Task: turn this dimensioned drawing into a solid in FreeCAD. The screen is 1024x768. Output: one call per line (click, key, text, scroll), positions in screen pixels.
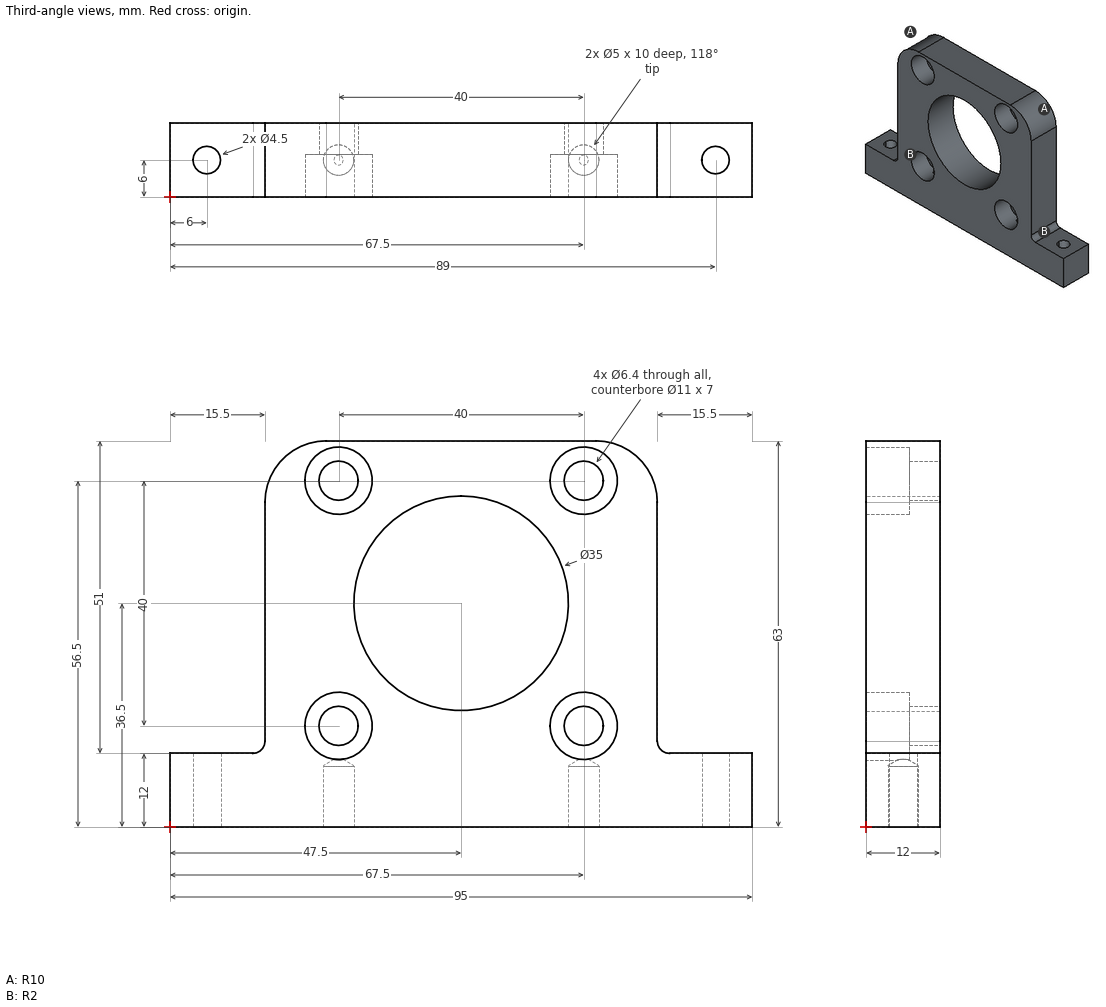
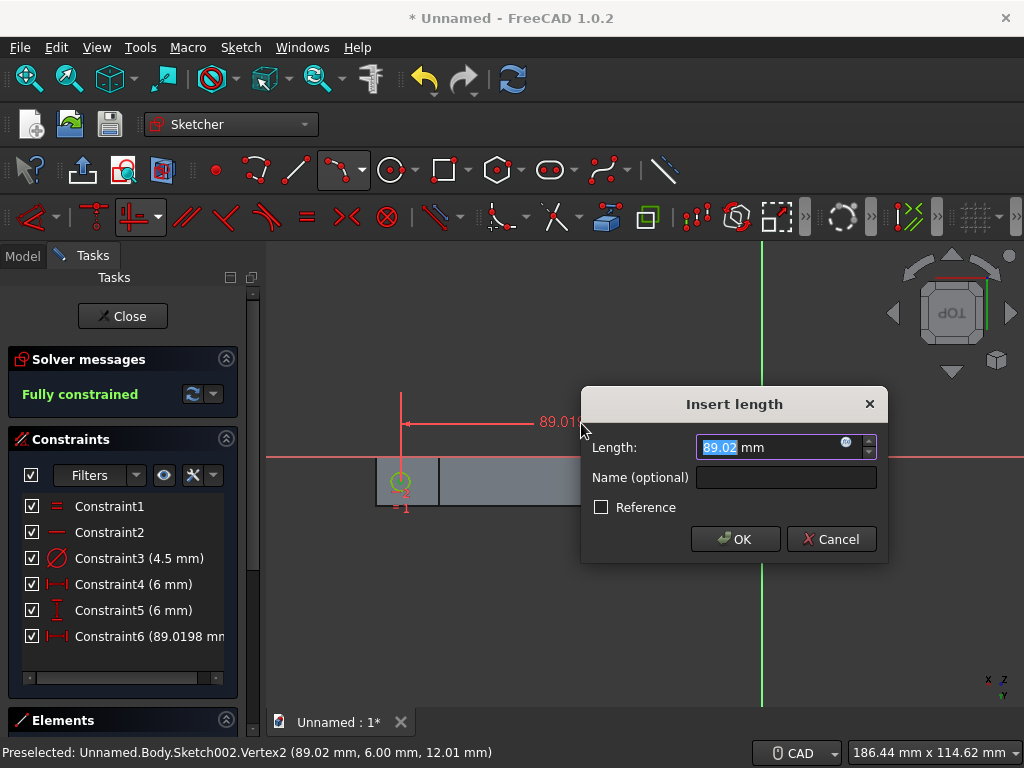
text(89)
key(Return)
key(Escape)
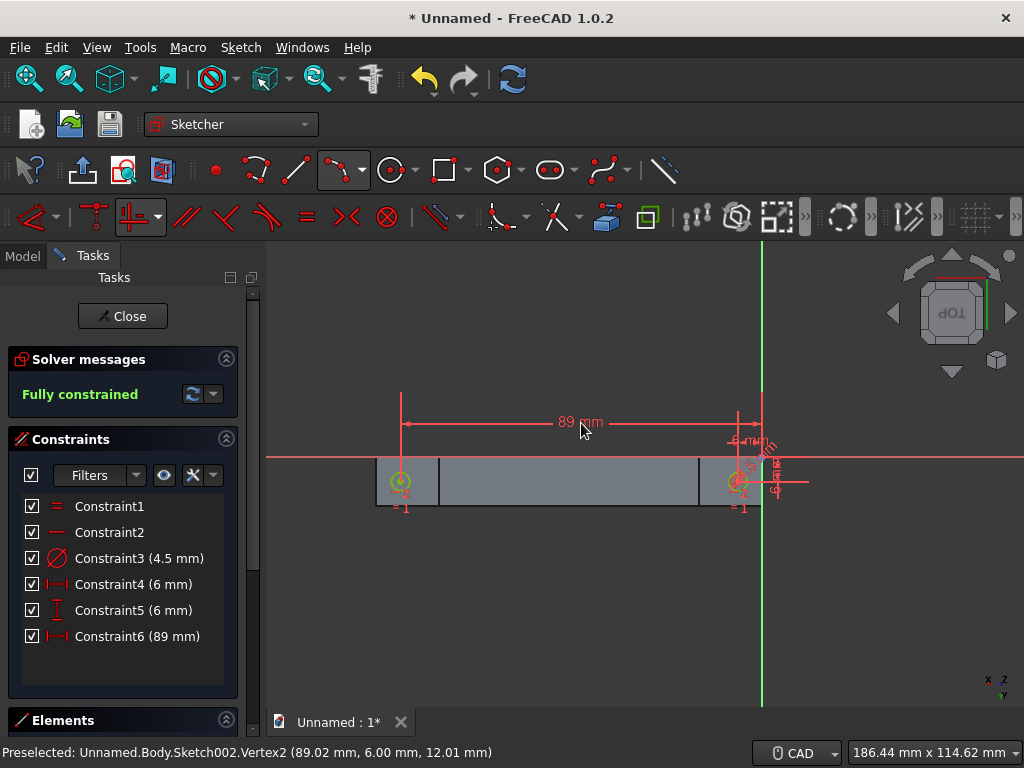
click(123, 316)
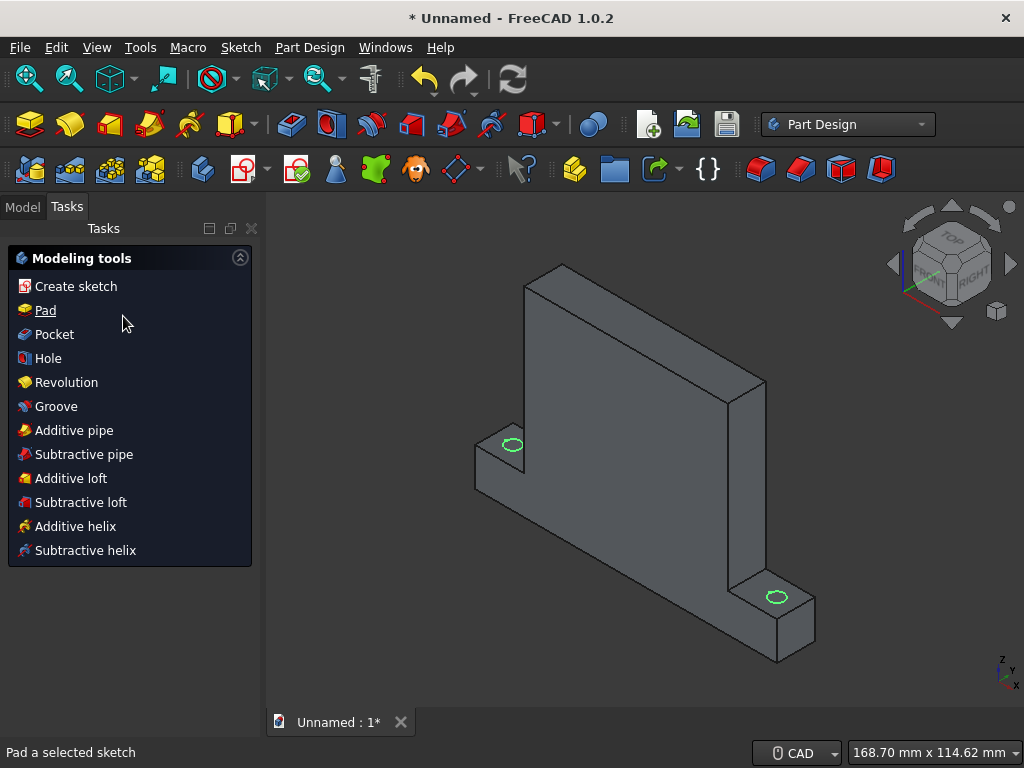
click(292, 124)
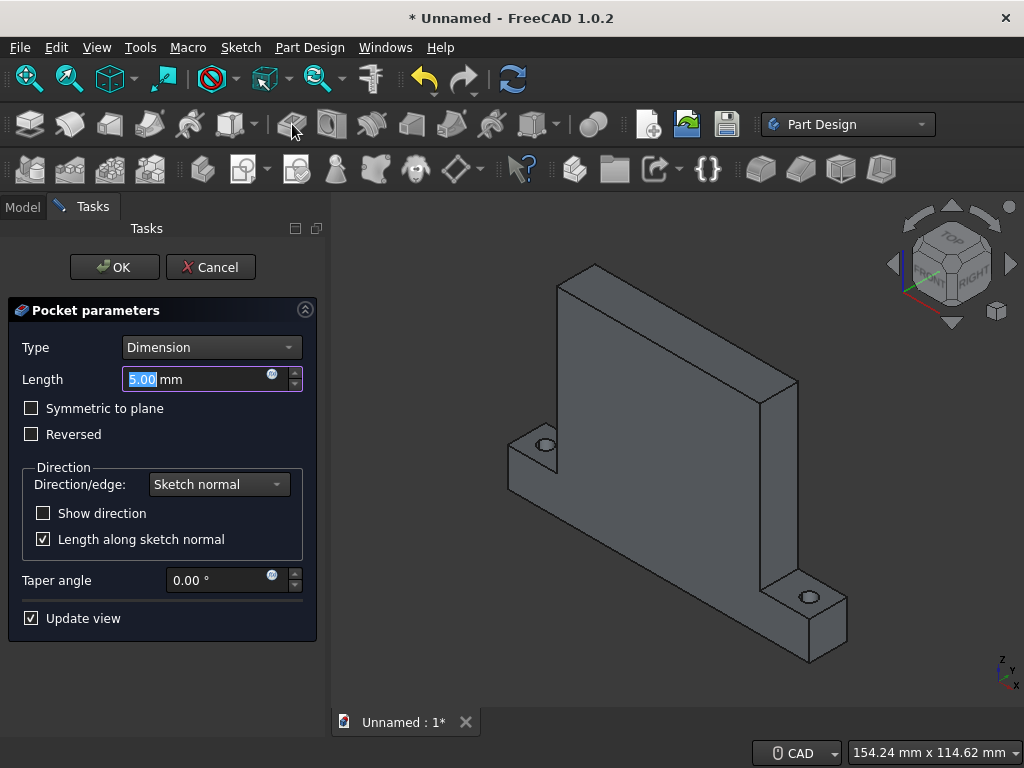
click(212, 348)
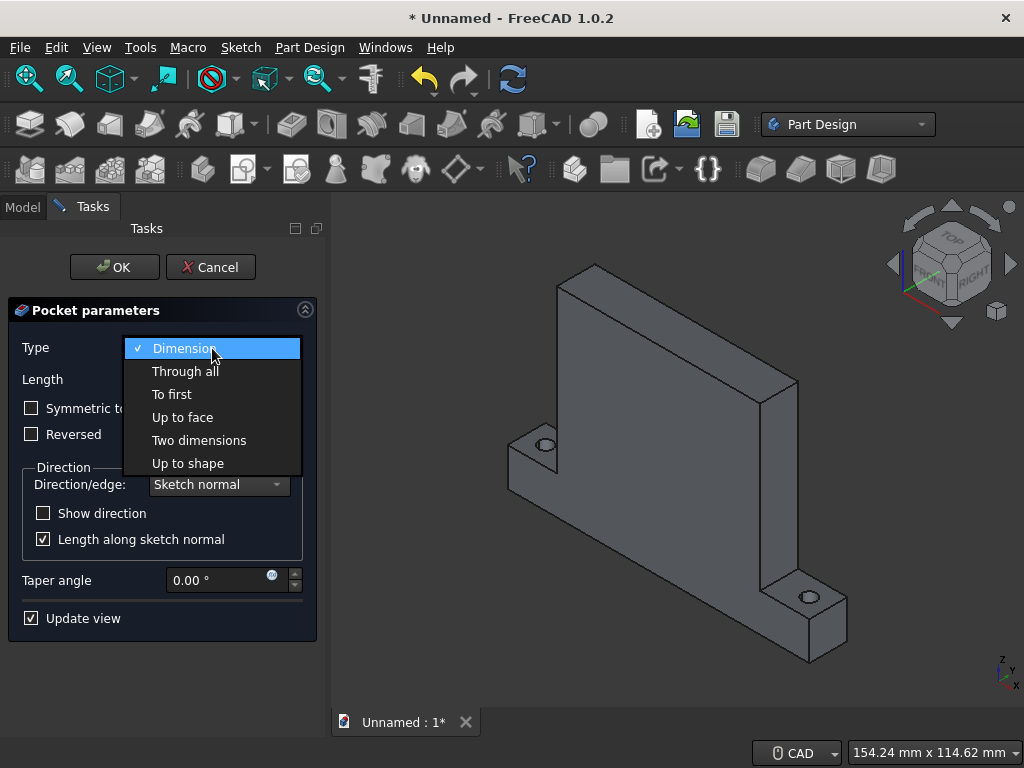
click(212, 372)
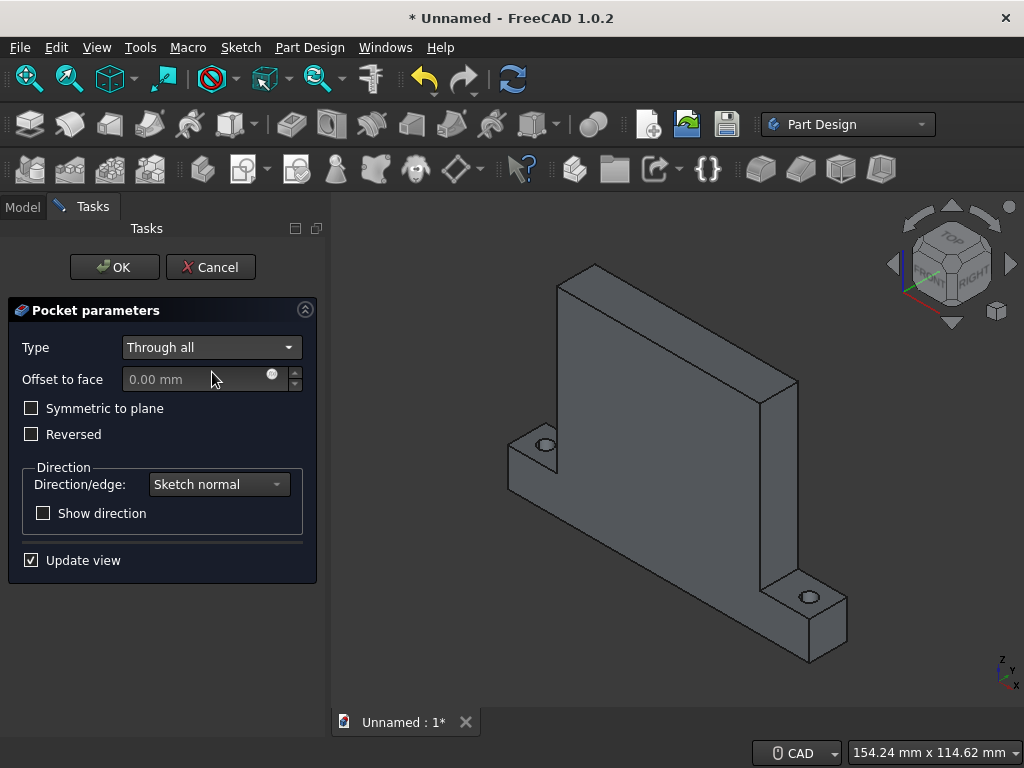
click(115, 267)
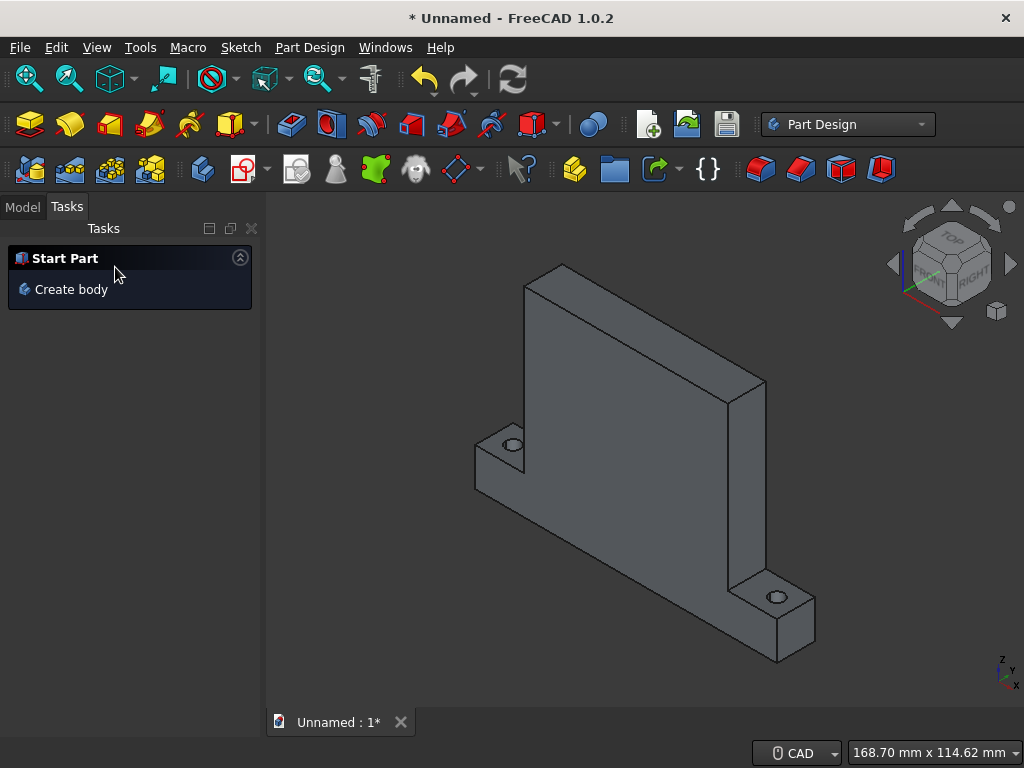
key(4)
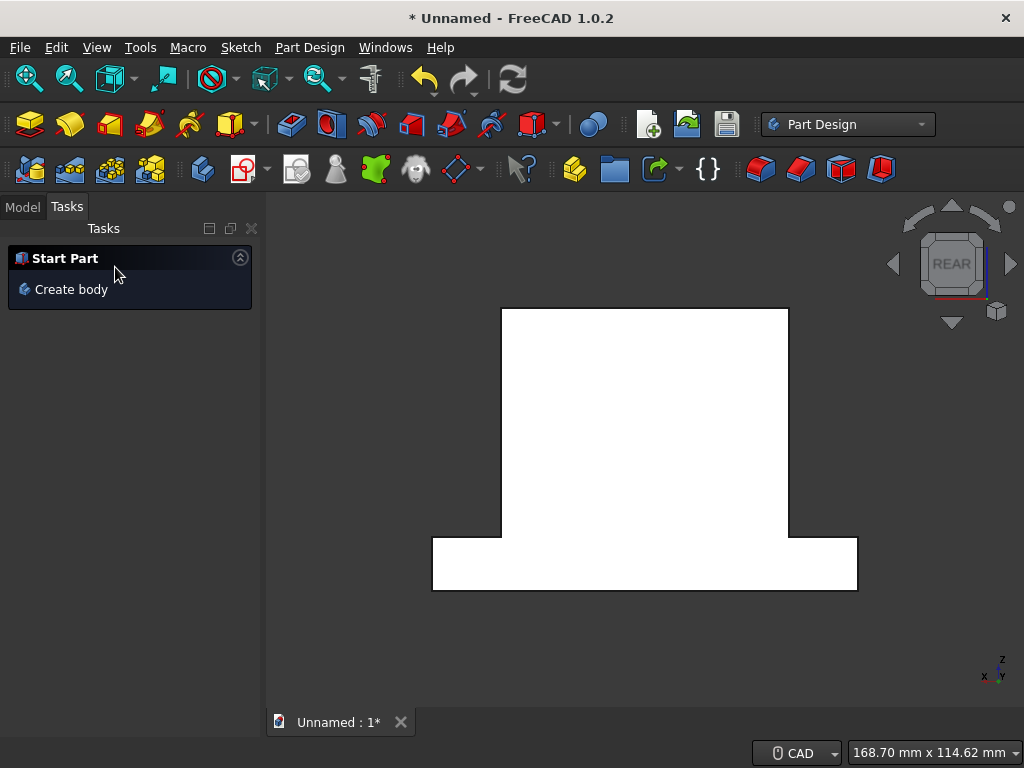
click(645, 449)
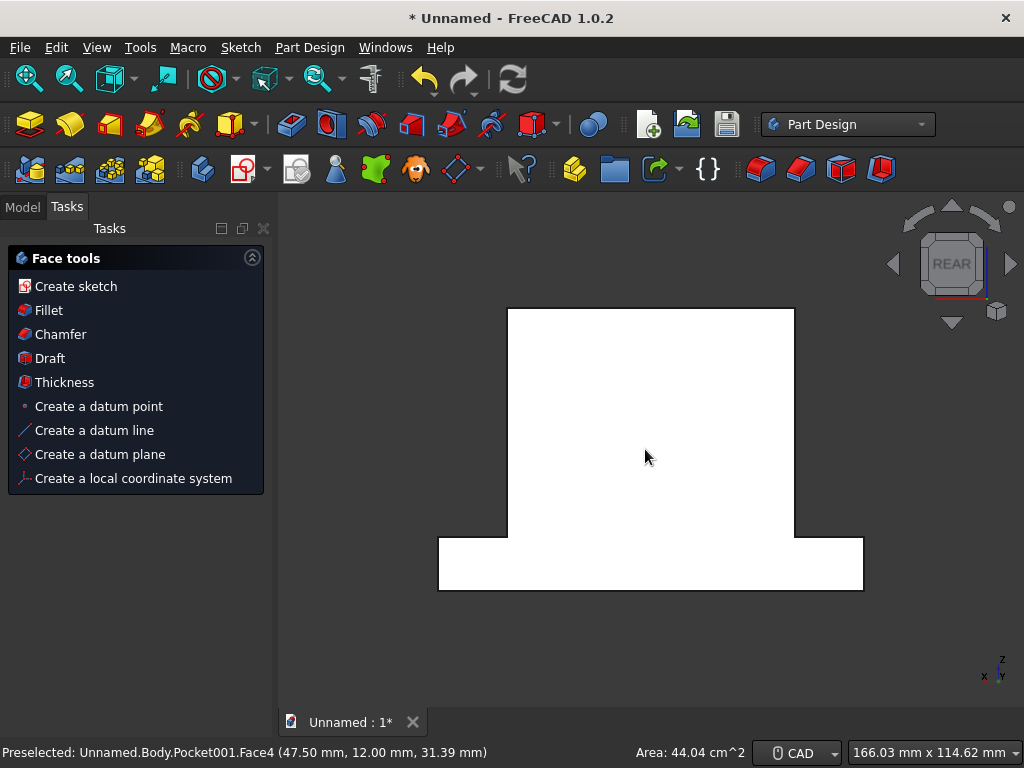
click(244, 170)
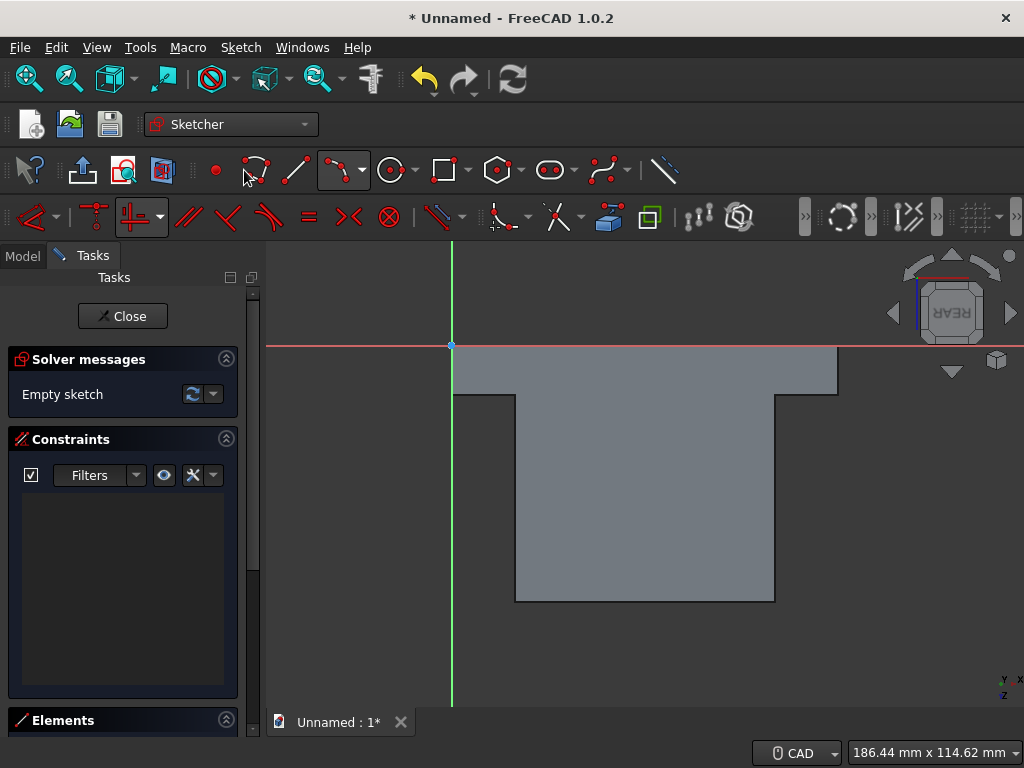
click(392, 170)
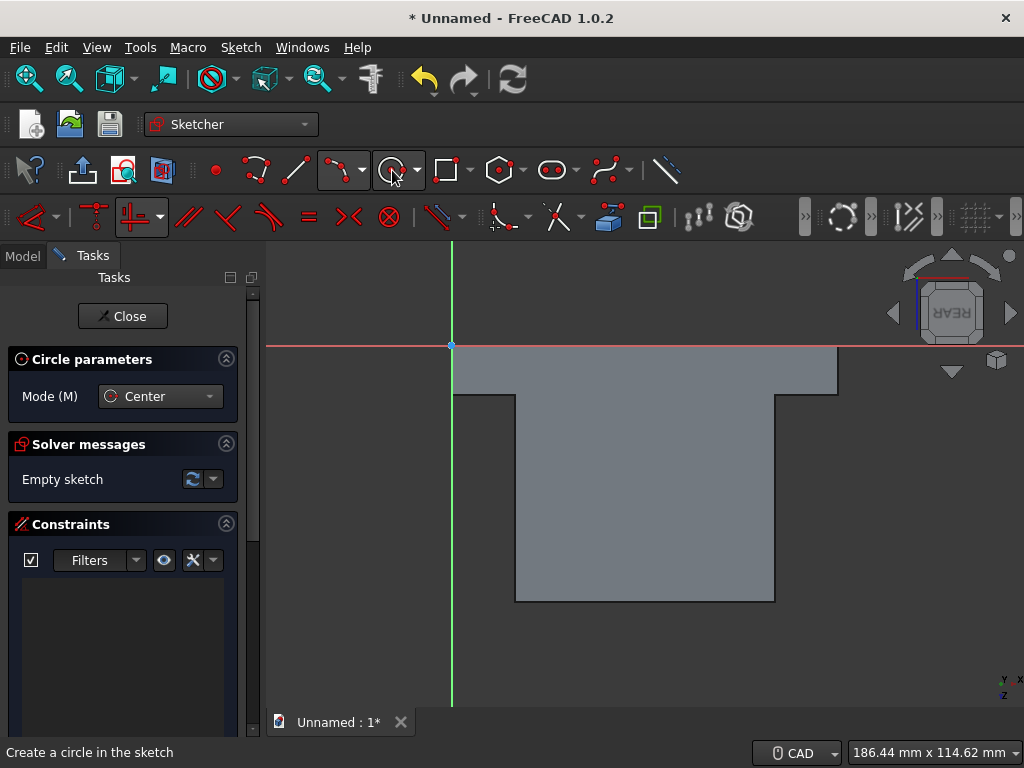
click(645, 494)
click(695, 444)
key(Escape)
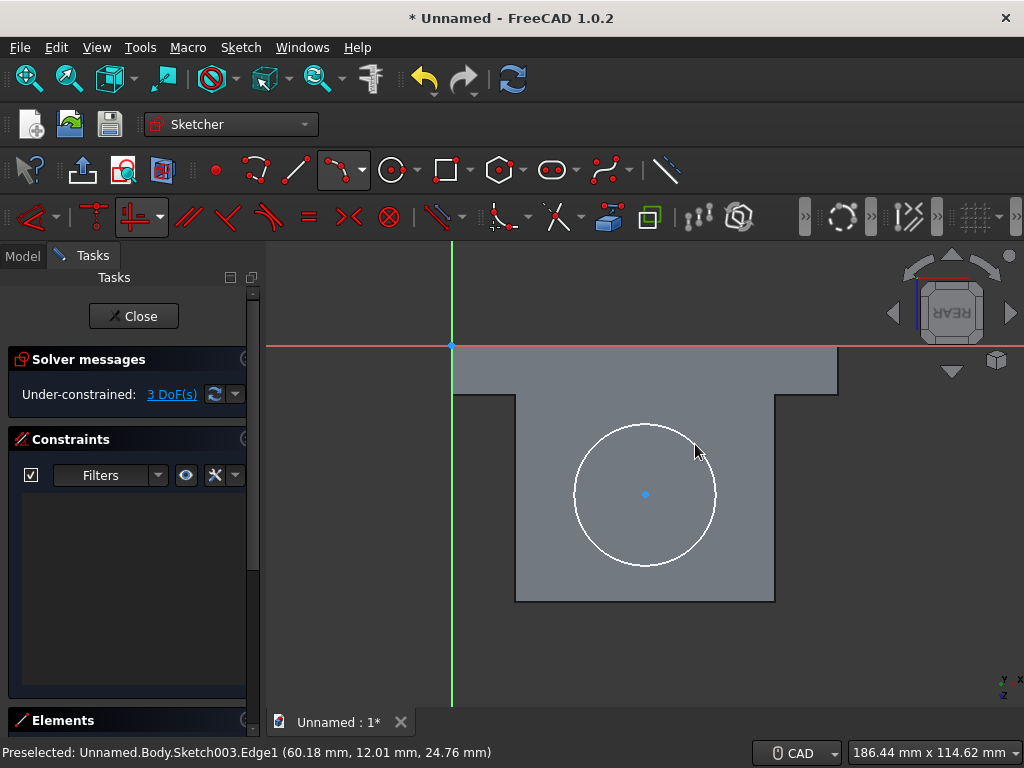
key(d)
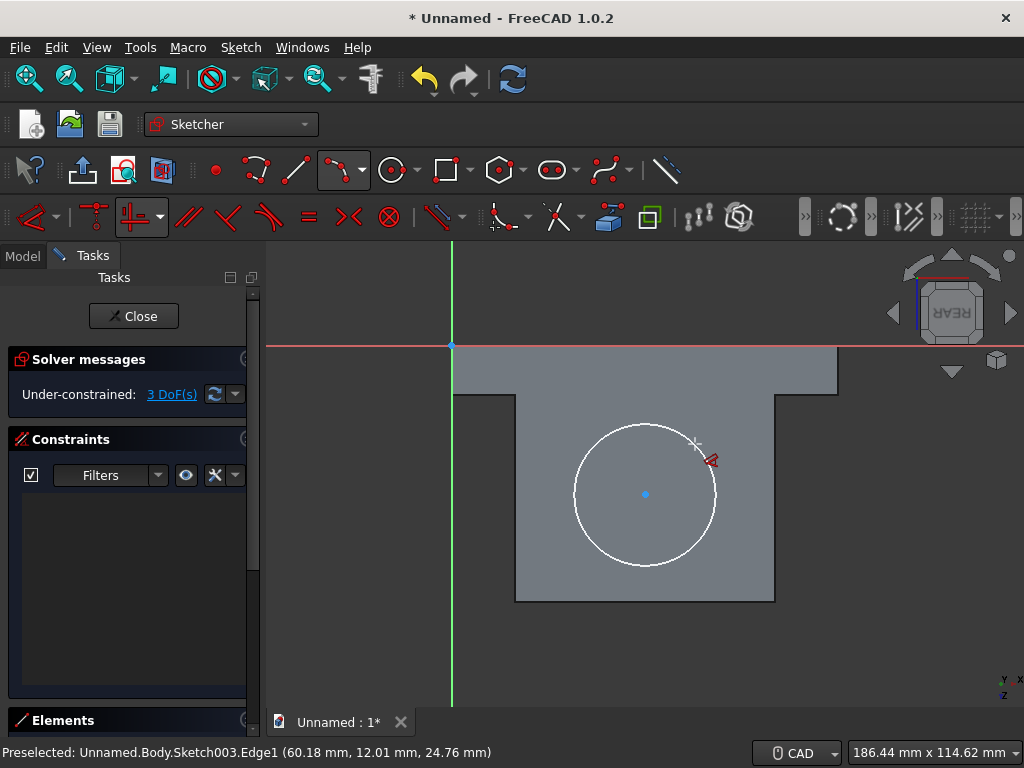
click(695, 445)
click(718, 422)